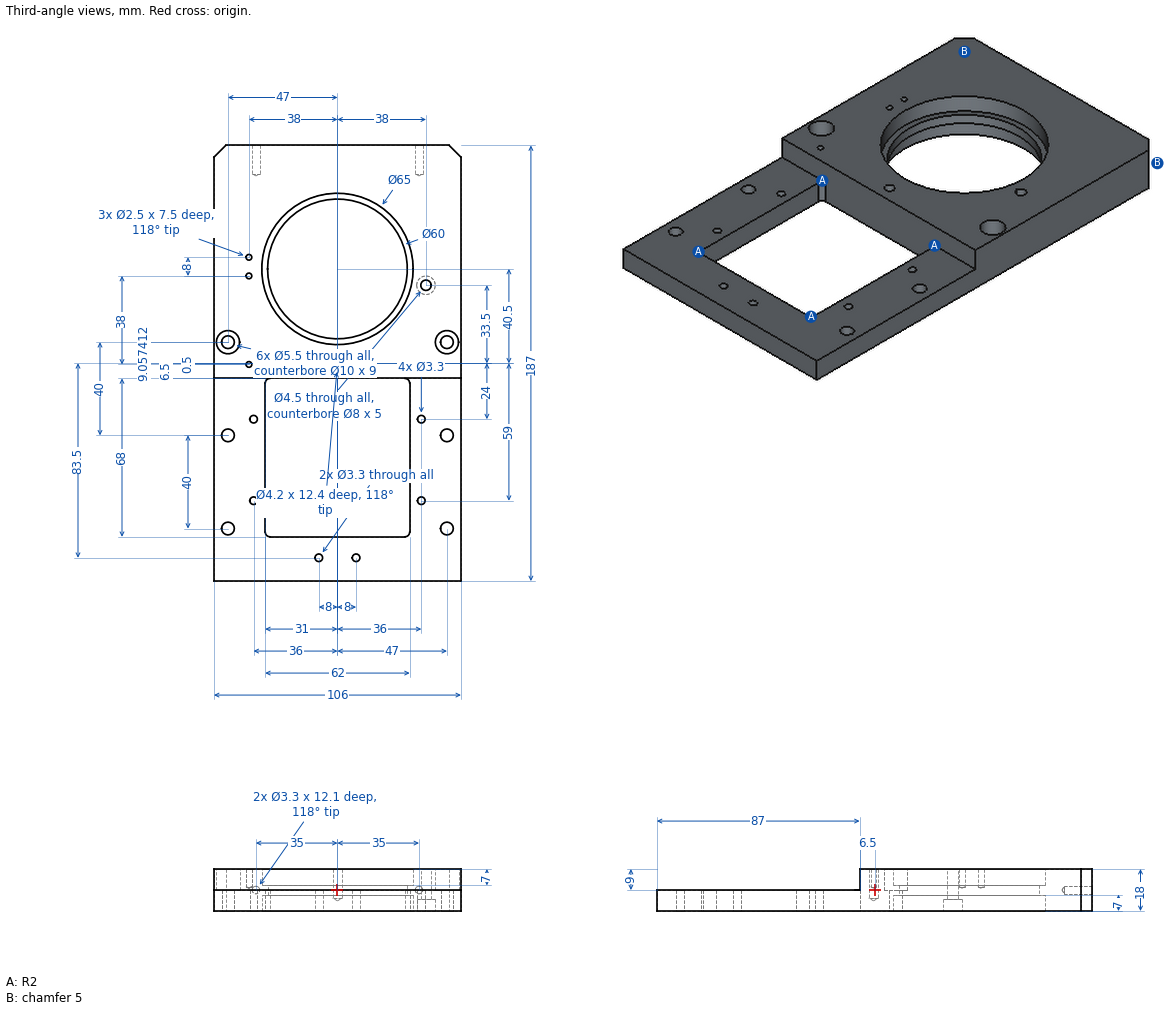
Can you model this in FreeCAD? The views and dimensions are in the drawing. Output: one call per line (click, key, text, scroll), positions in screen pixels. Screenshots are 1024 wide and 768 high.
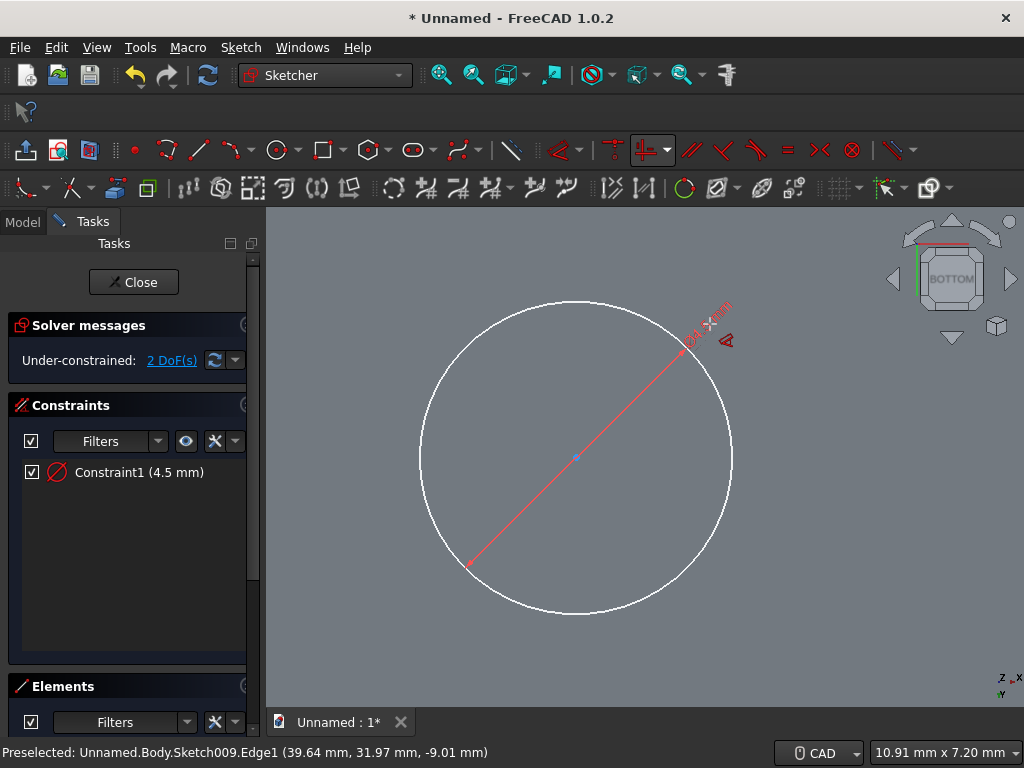
click(576, 458)
click(370, 492)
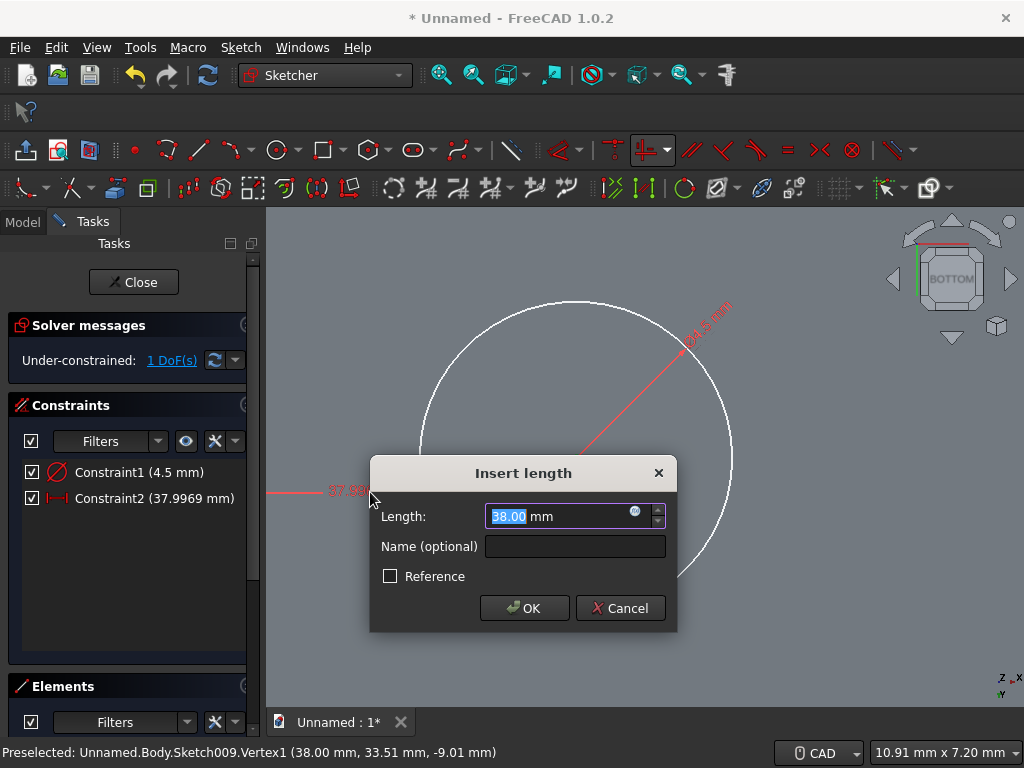
text(38)
key(Return)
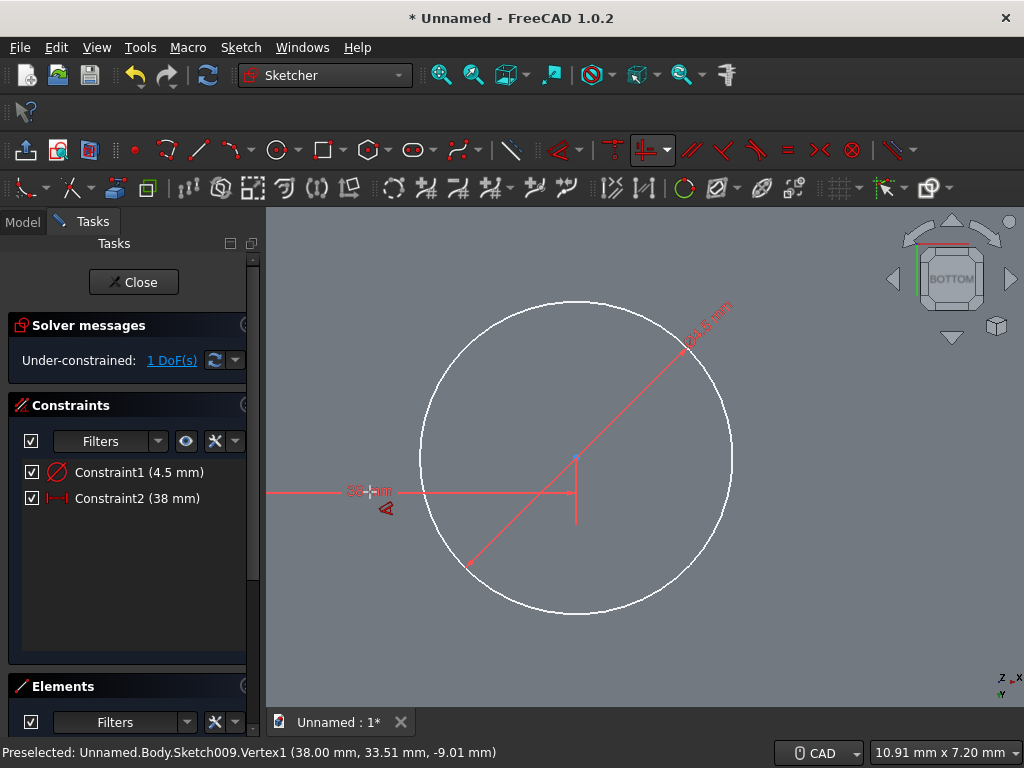
click(576, 458)
click(610, 346)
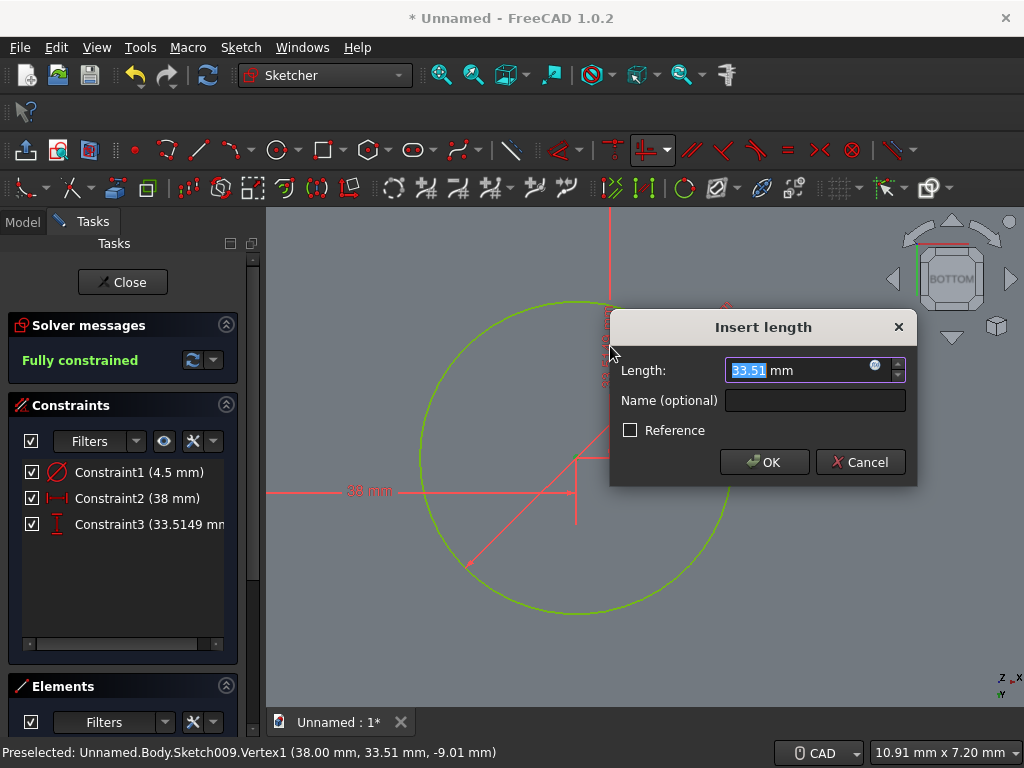
text(33.5)
key(Return)
key(Escape)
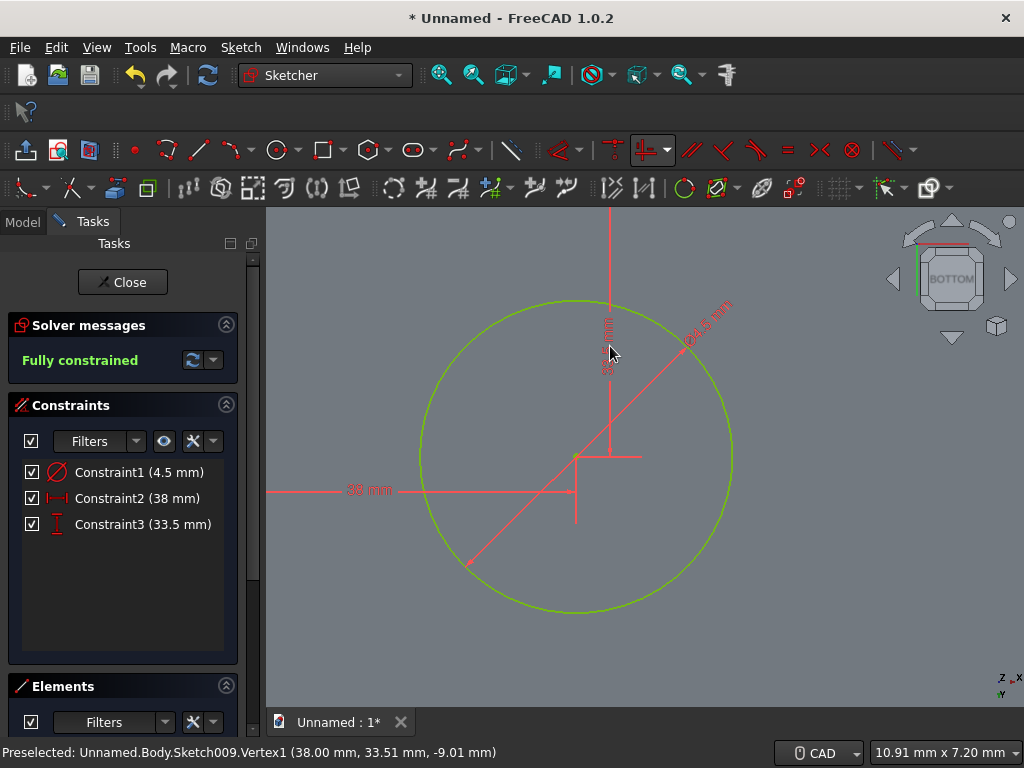
click(123, 282)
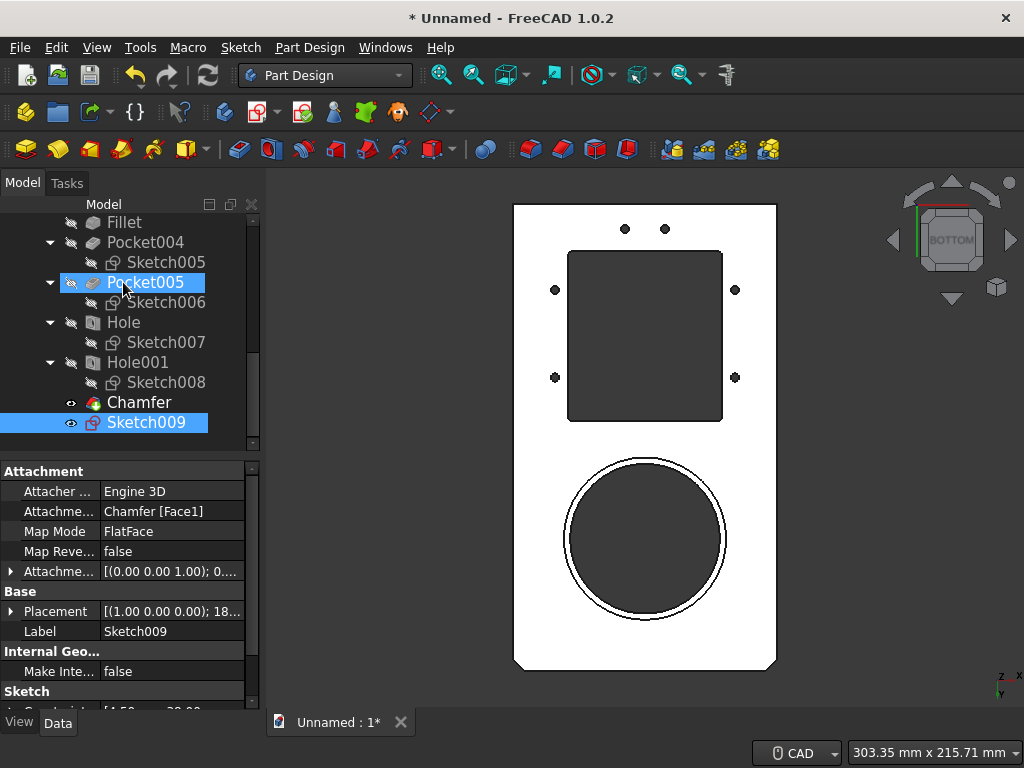
click(272, 150)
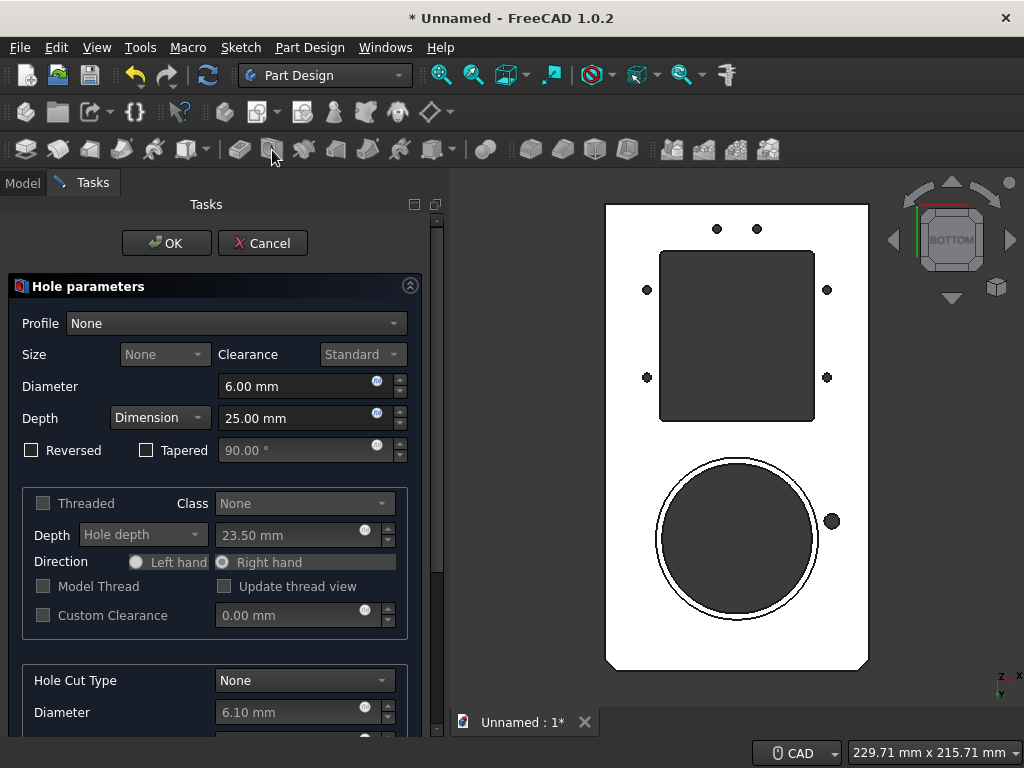
triple_click(305, 386)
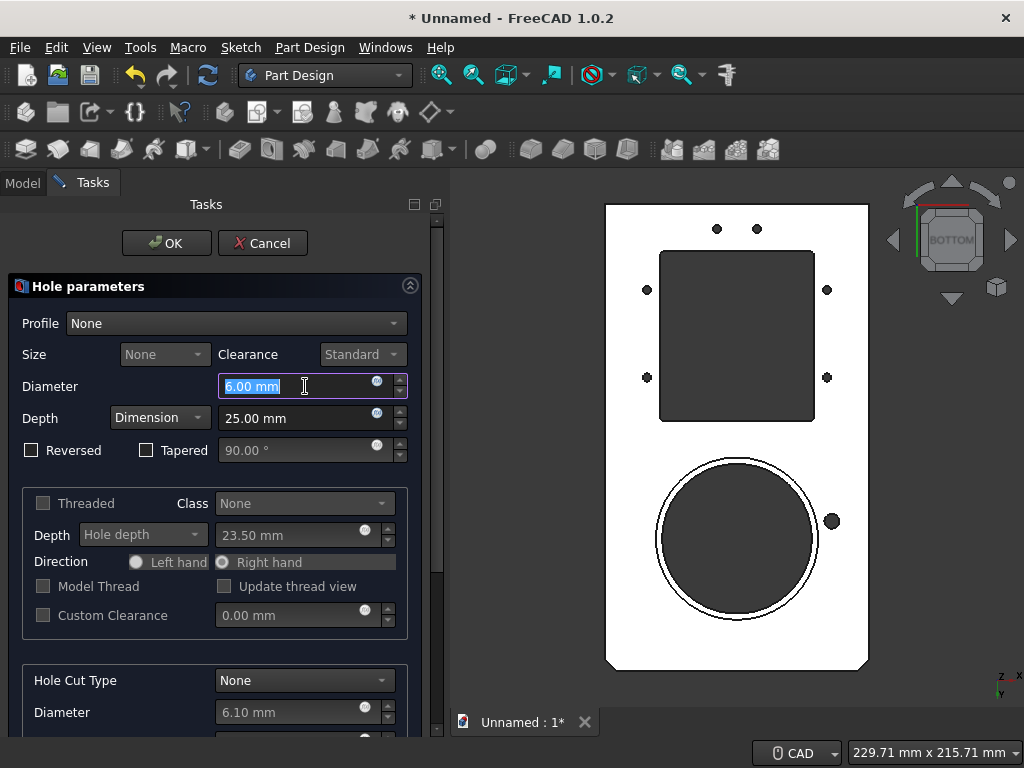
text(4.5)
key(Tab)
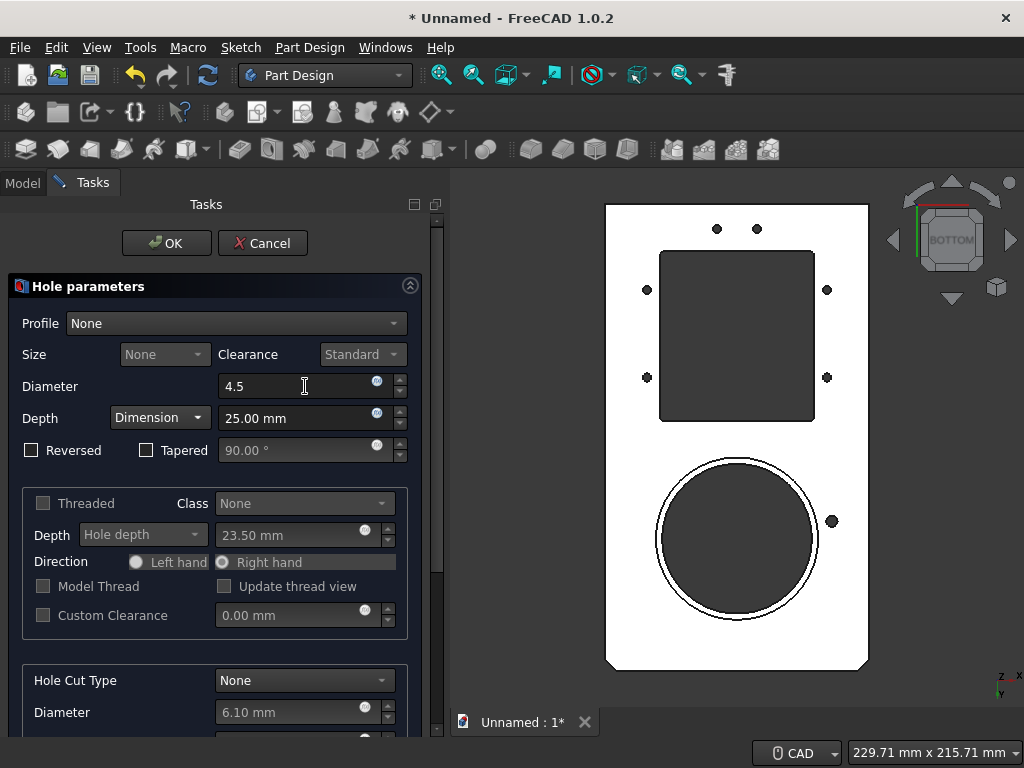
click(161, 418)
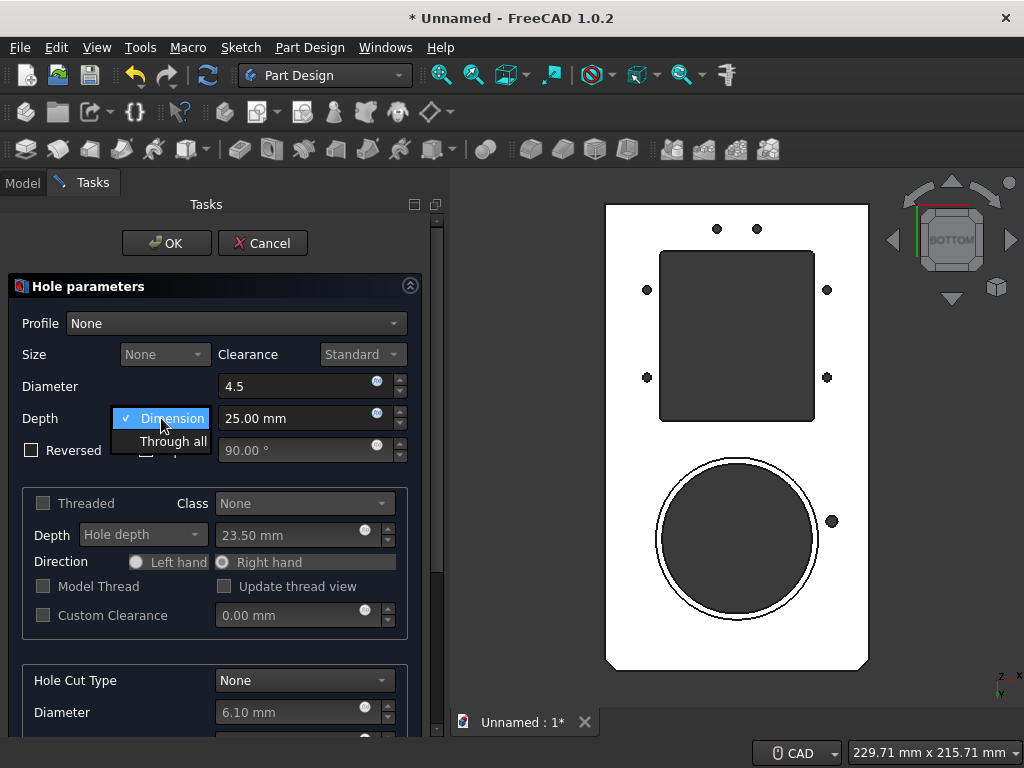
click(160, 442)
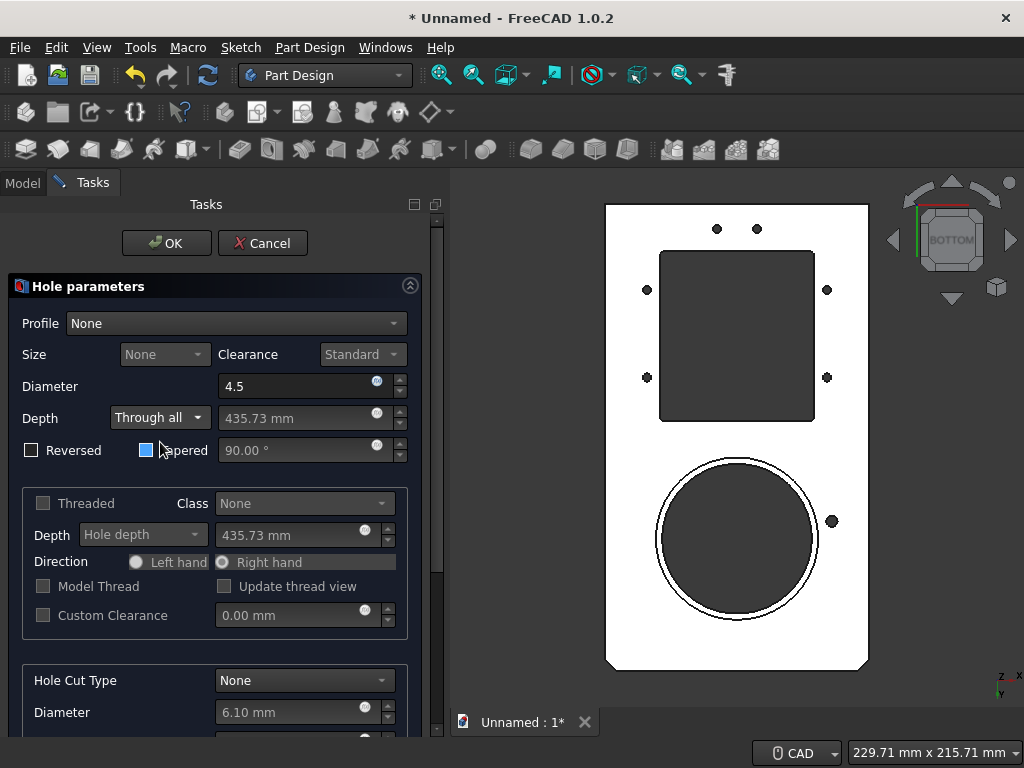
click(306, 680)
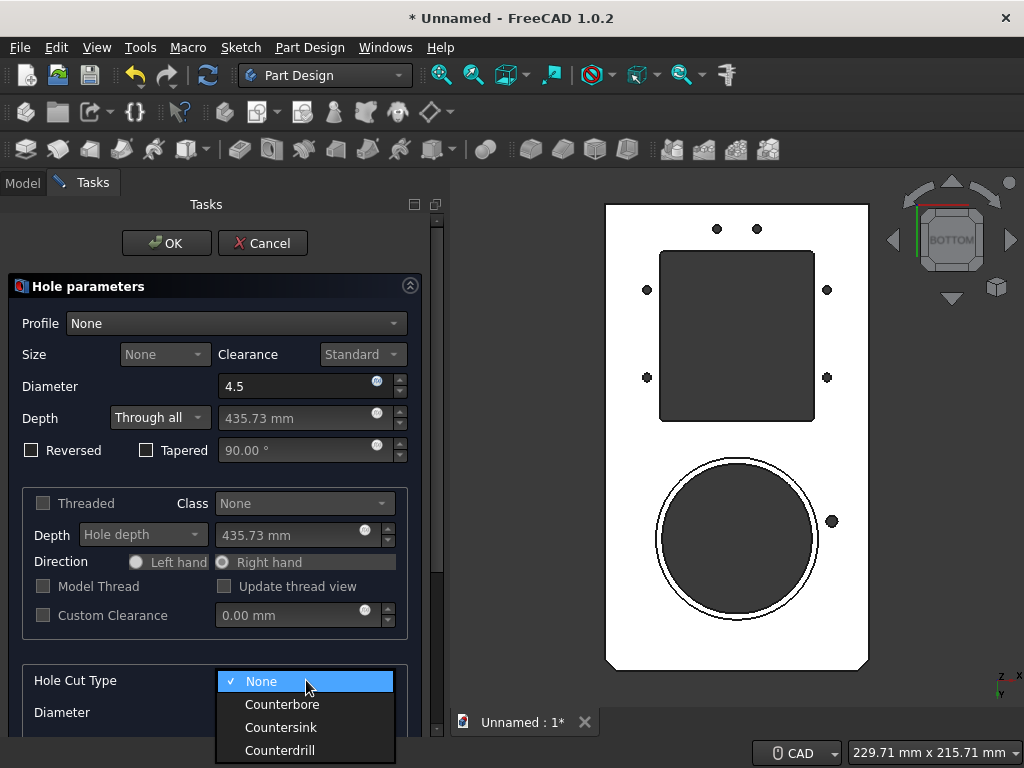
click(304, 704)